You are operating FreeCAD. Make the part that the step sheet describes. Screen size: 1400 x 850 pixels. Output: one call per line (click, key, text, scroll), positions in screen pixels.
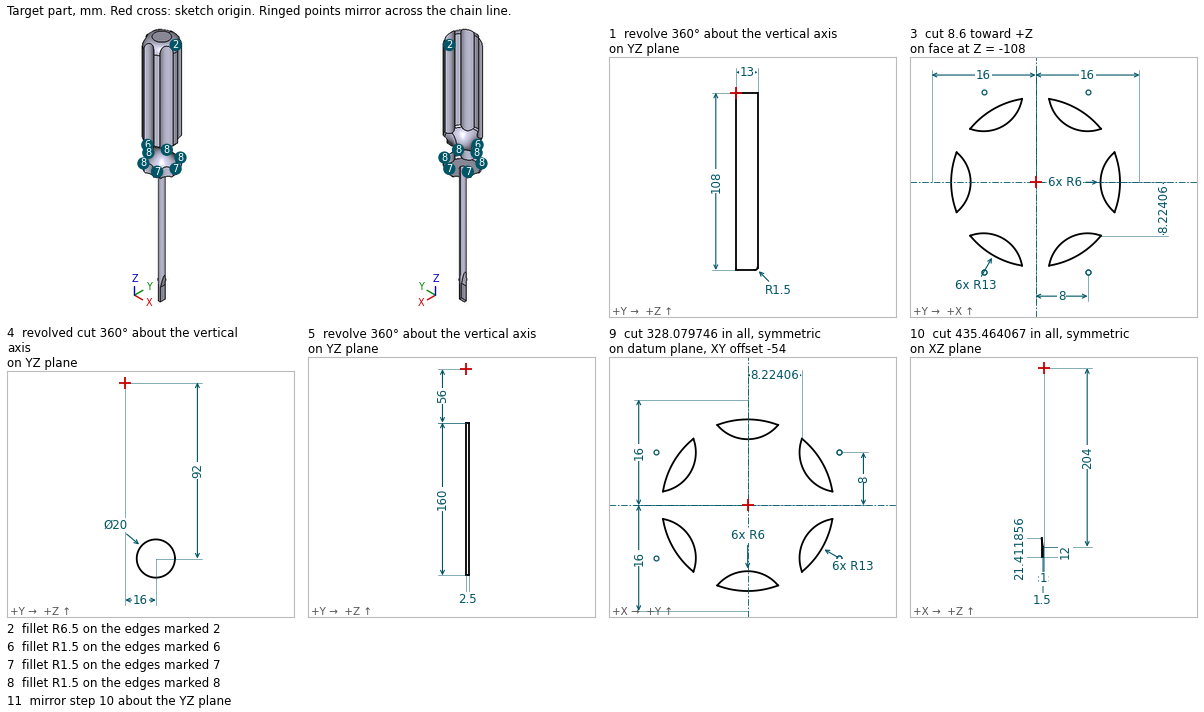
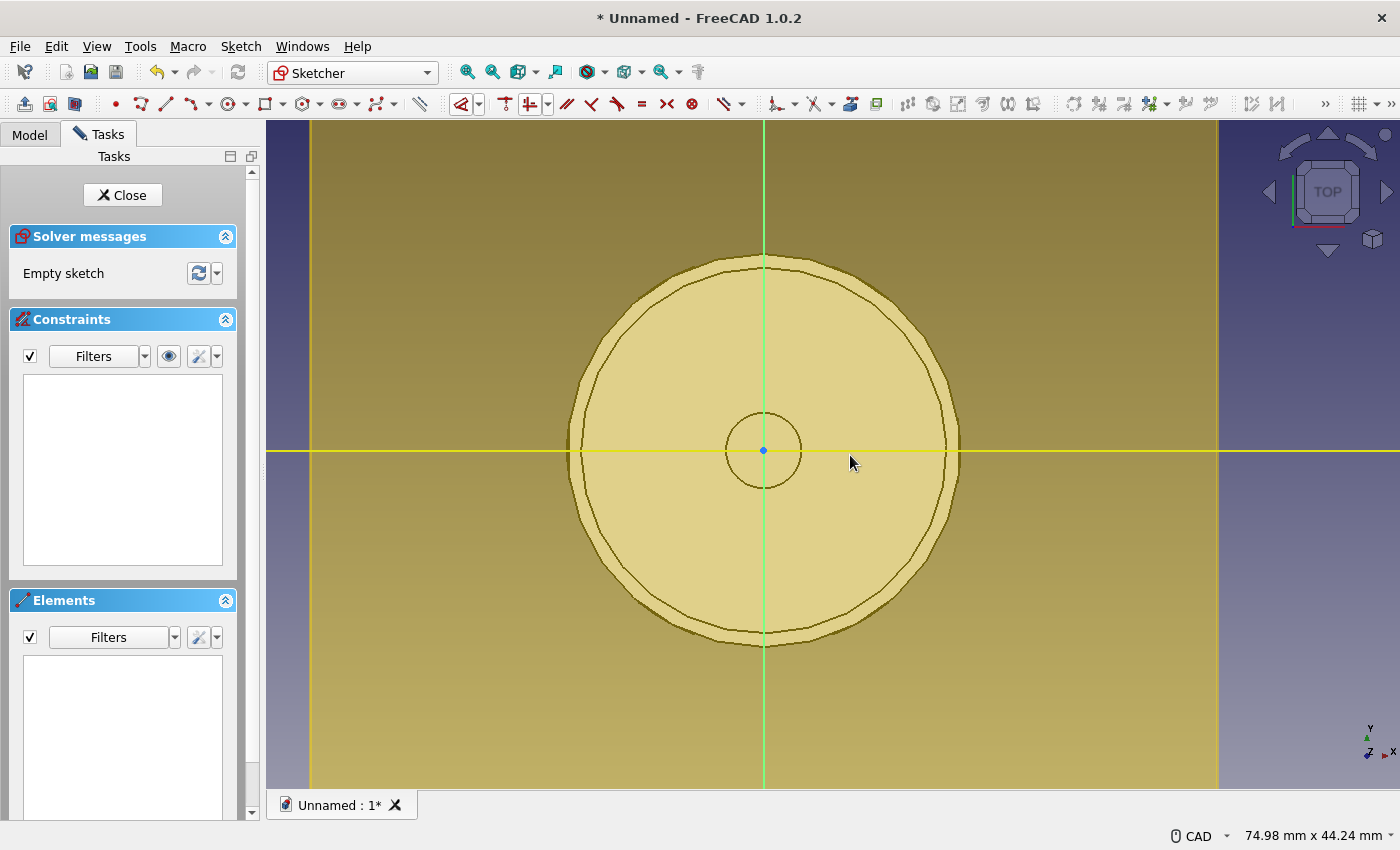
key(g)
key(3)
key(a)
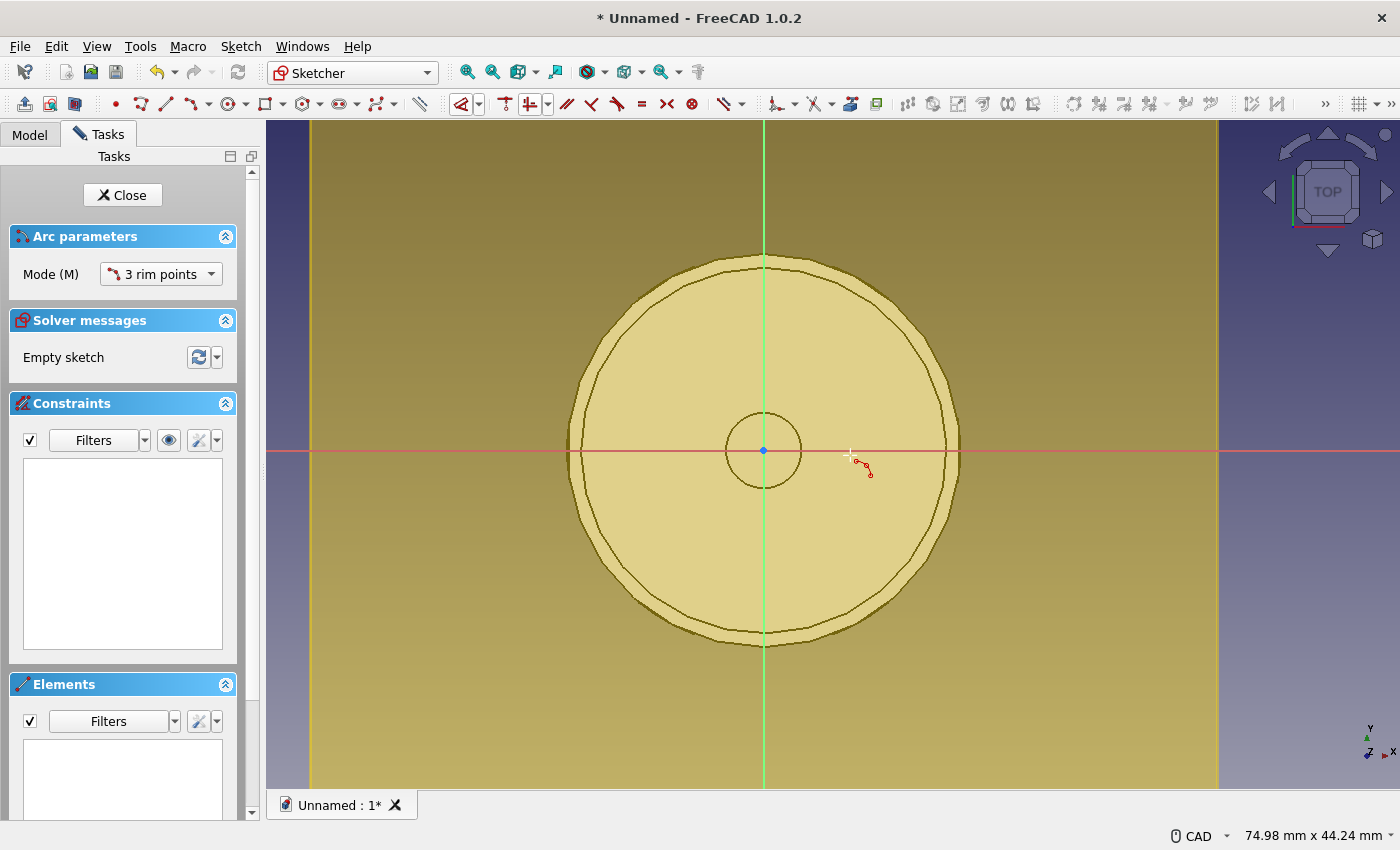
click(958, 419)
click(888, 298)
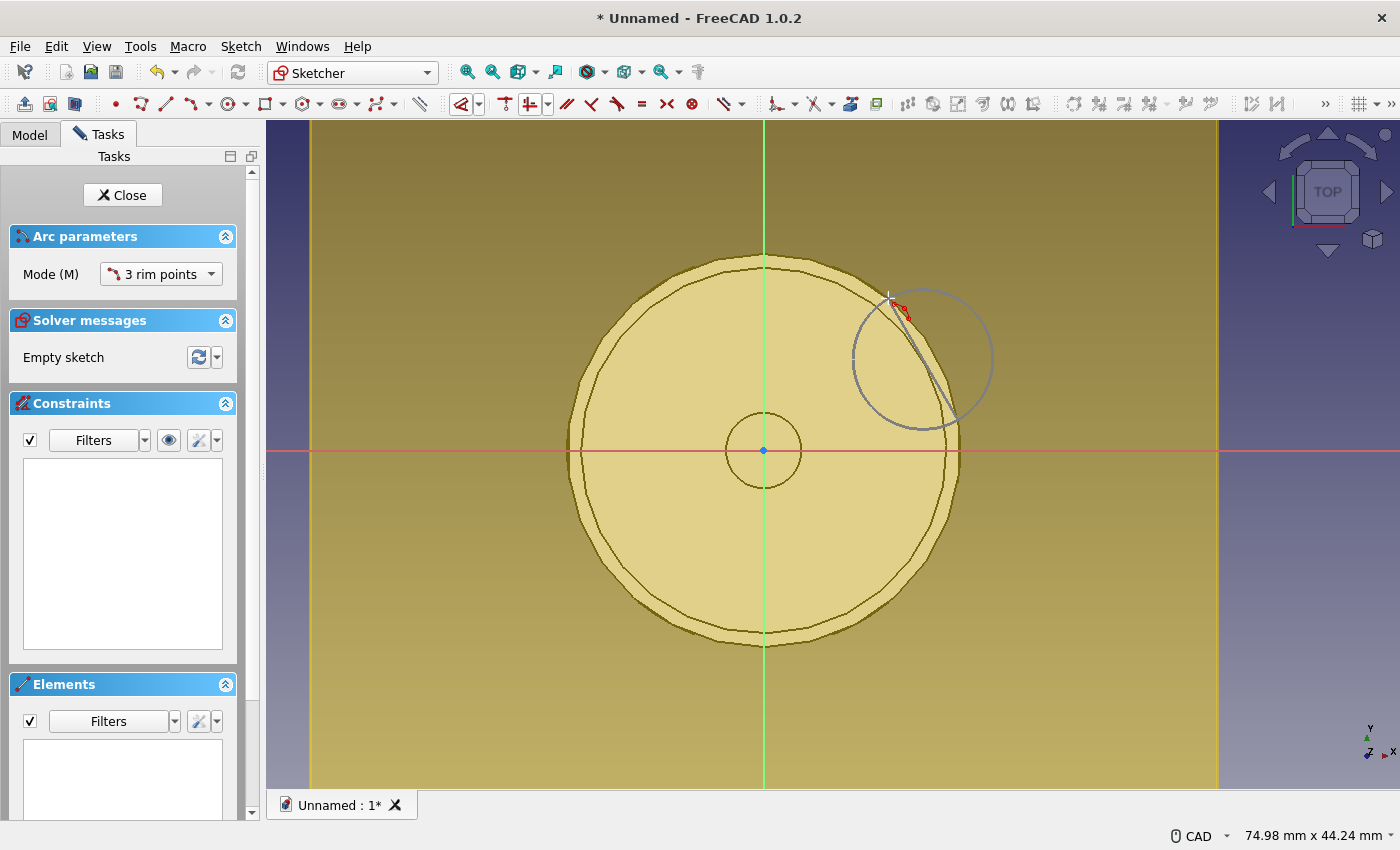
scroll(934, 352, up, 2)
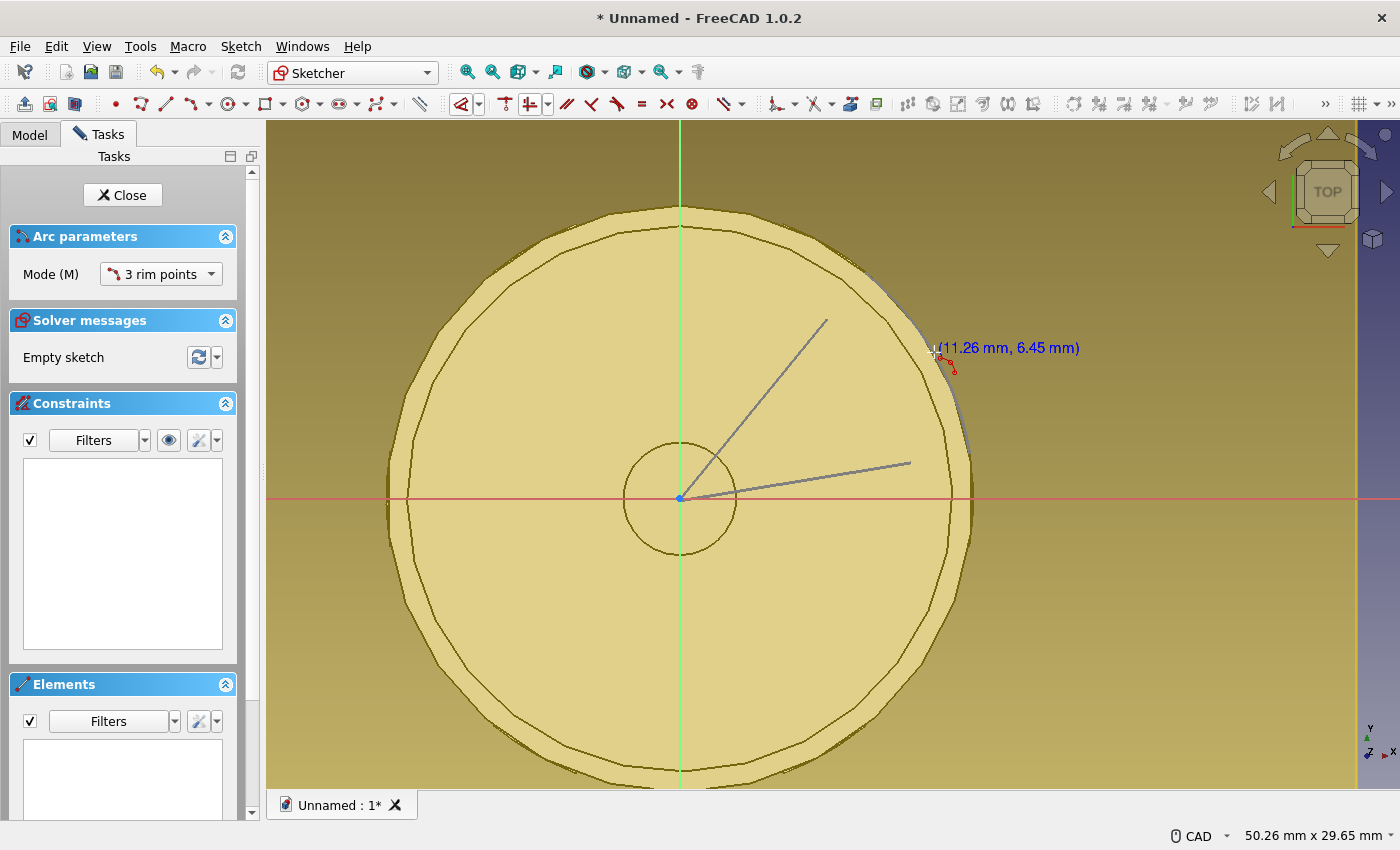
click(934, 352)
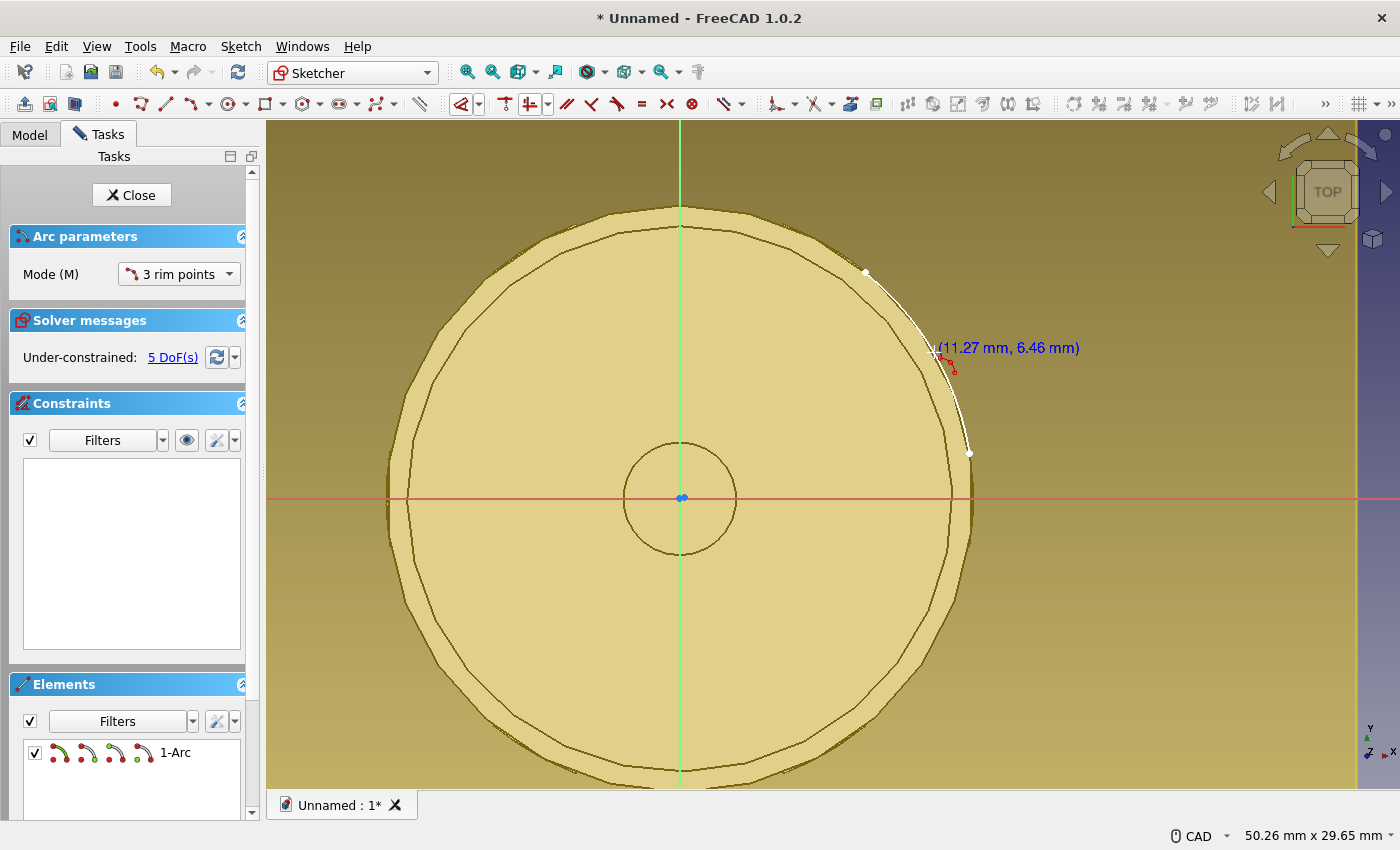
click(865, 273)
click(970, 453)
click(875, 386)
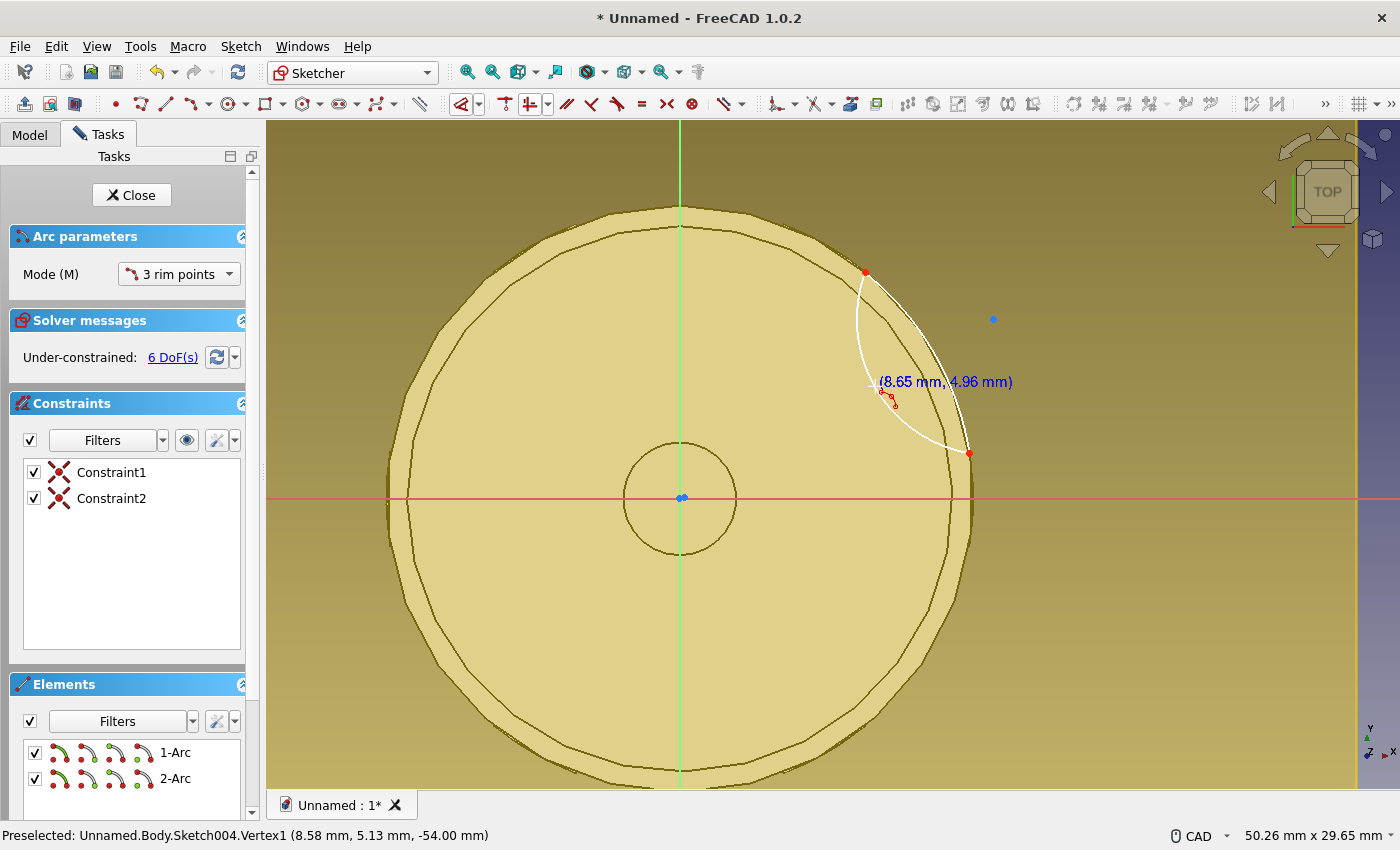
click(969, 546)
click(865, 726)
click(875, 612)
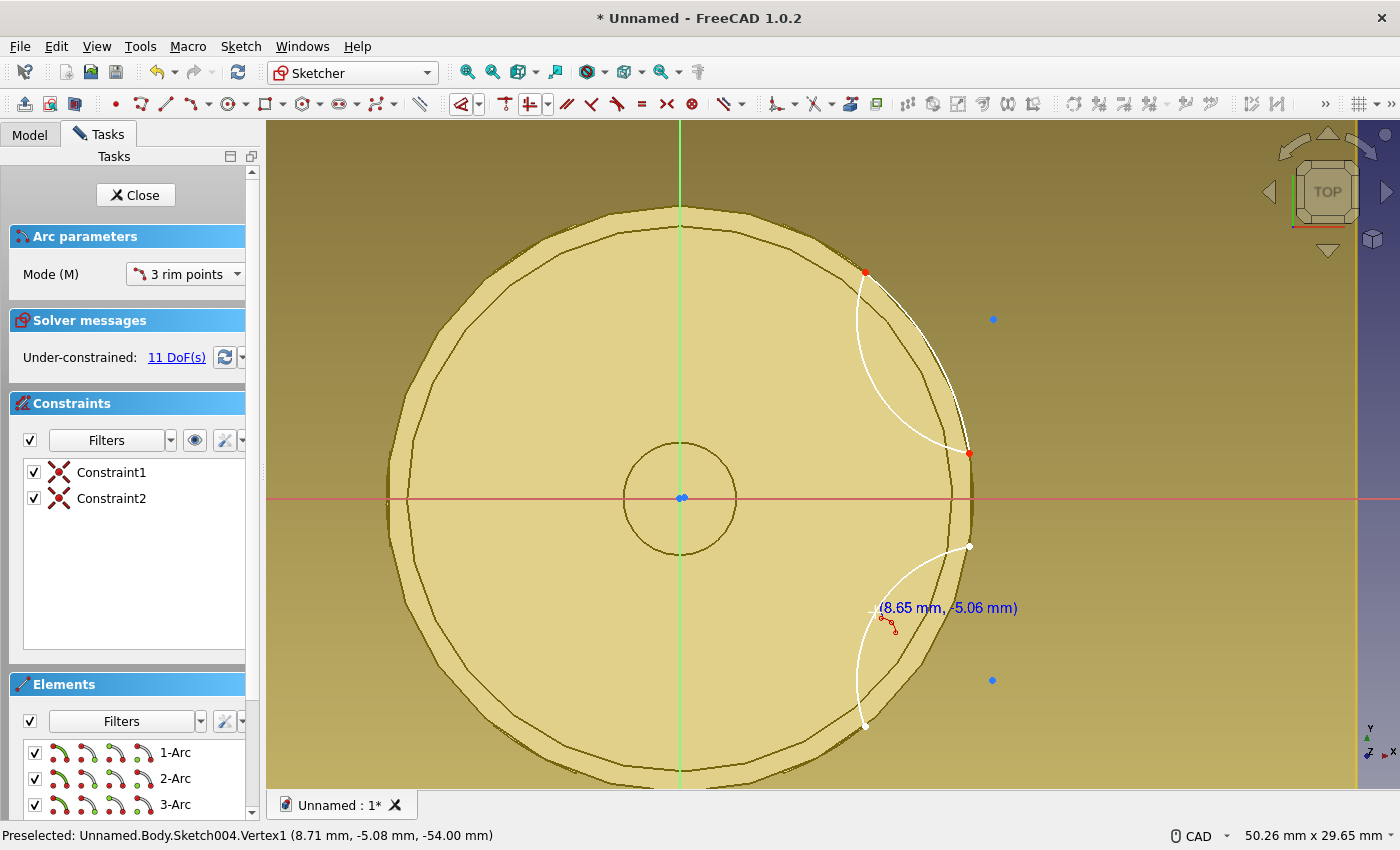
click(865, 727)
click(969, 547)
click(934, 645)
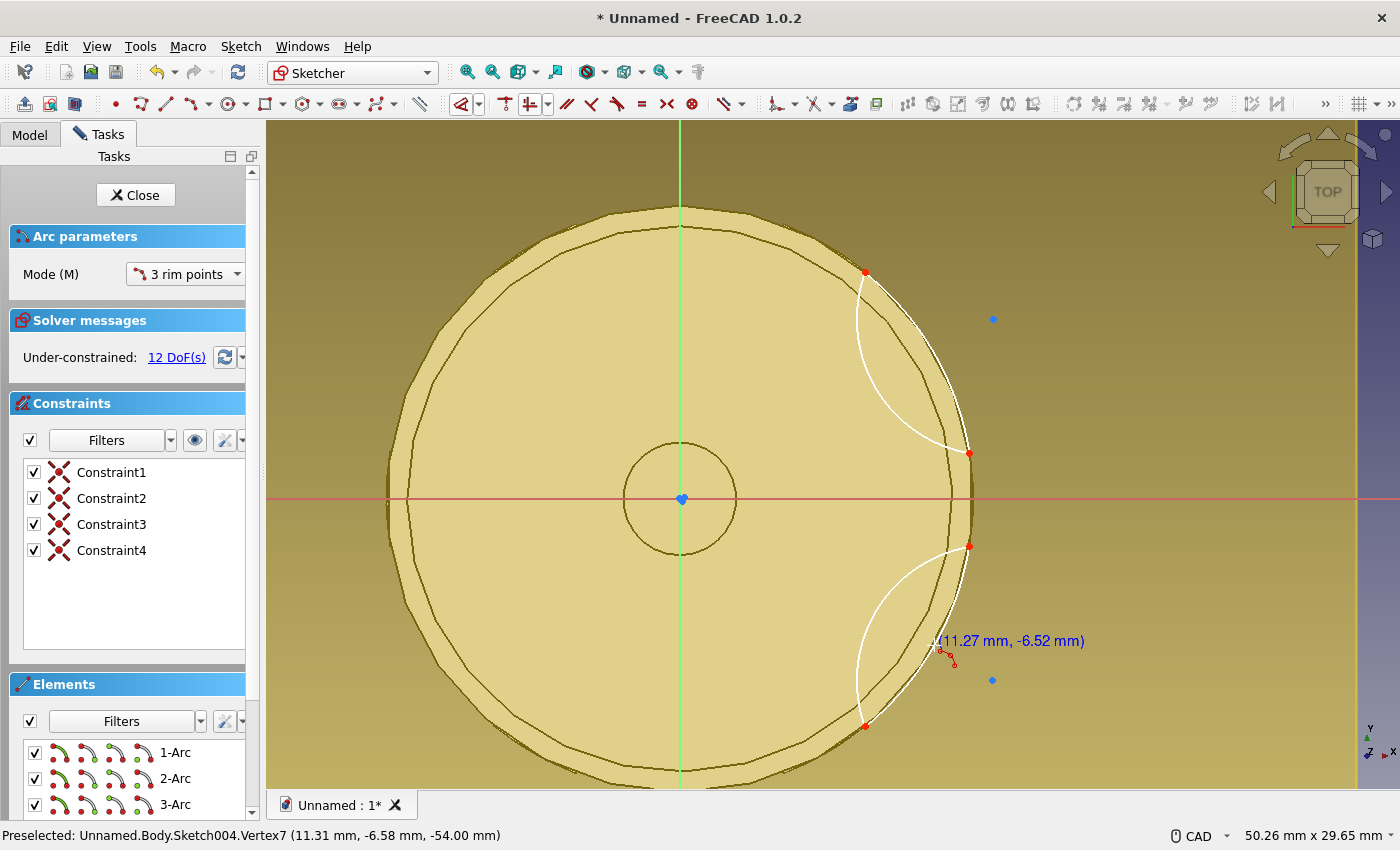
scroll(937, 364, down, 2)